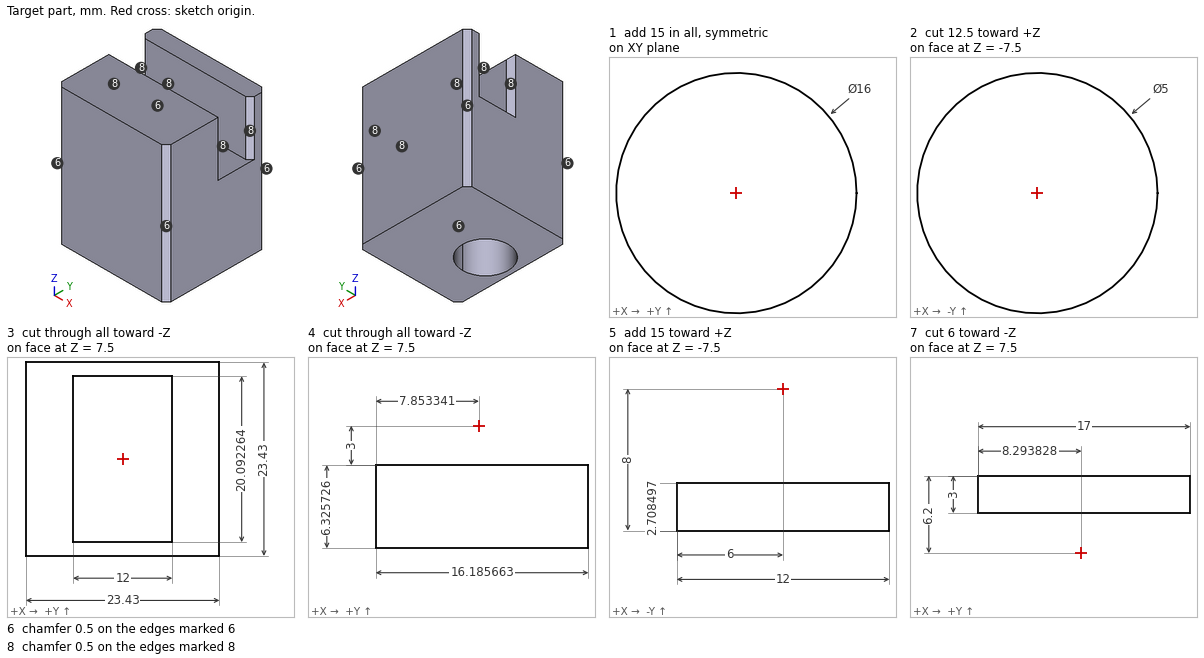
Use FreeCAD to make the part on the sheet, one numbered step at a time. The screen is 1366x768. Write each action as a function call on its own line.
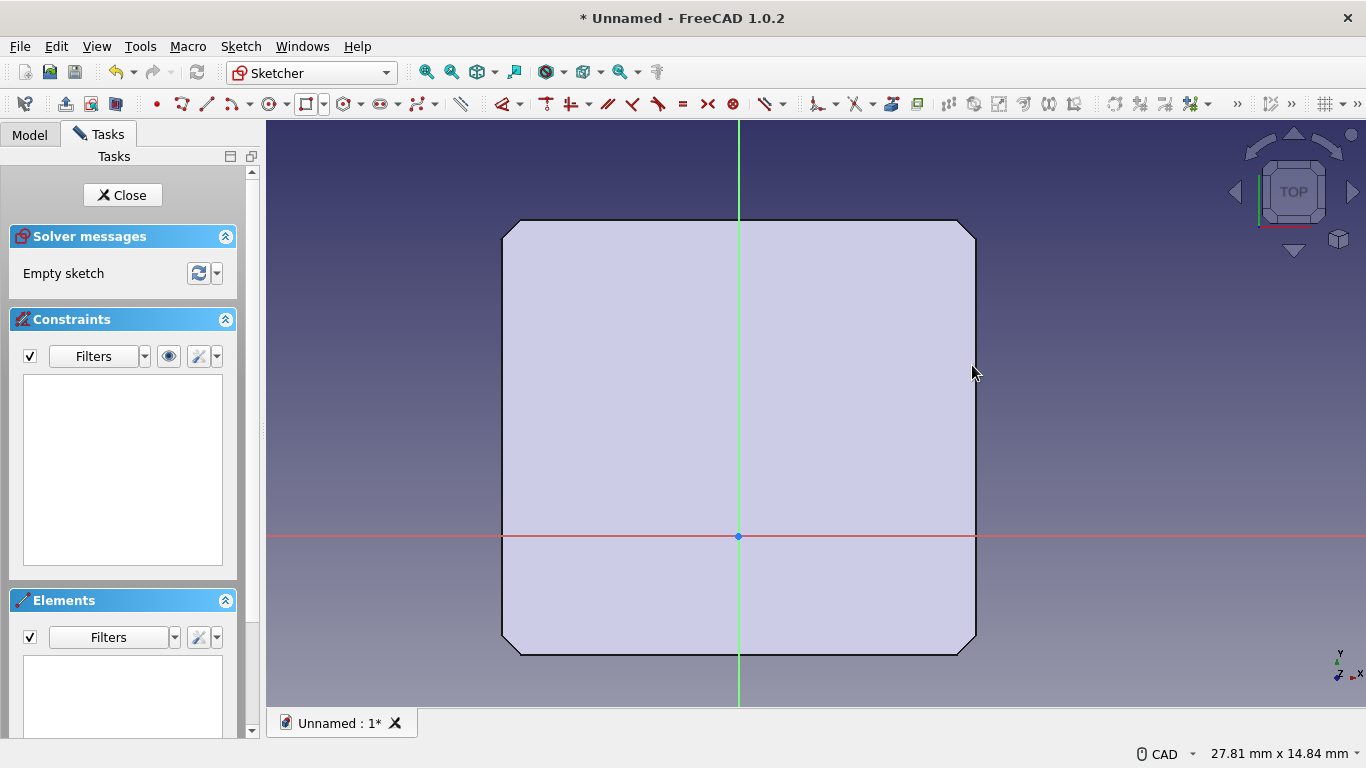
click(306, 104)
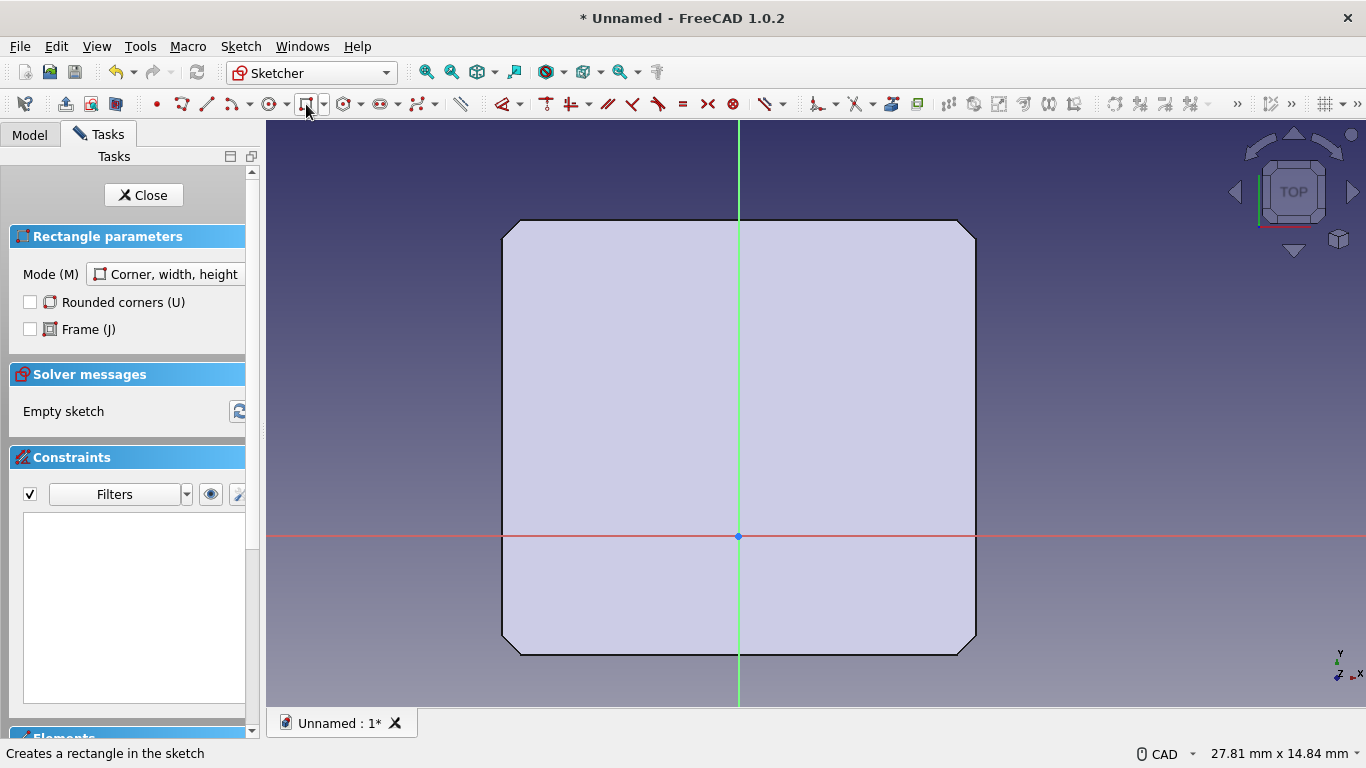
click(411, 291)
click(1083, 409)
key(Escape)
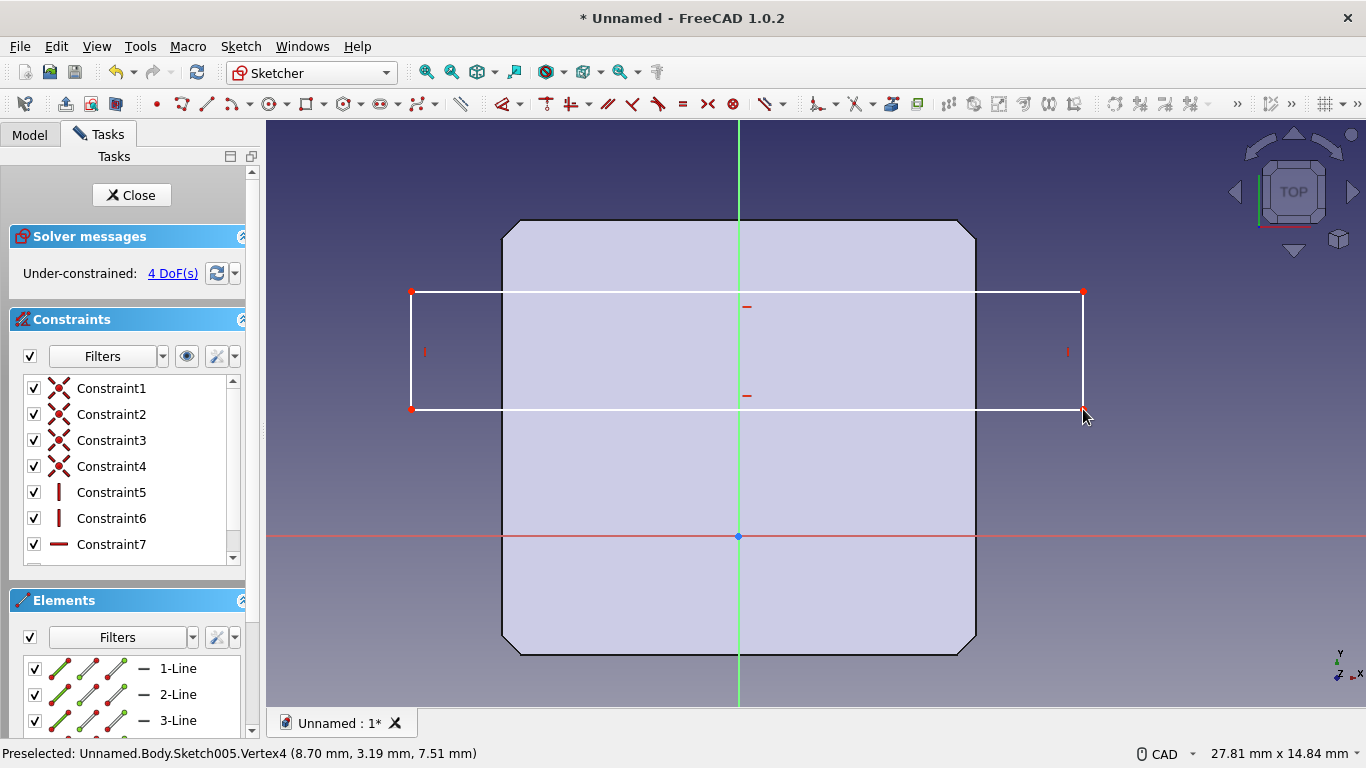
click(502, 104)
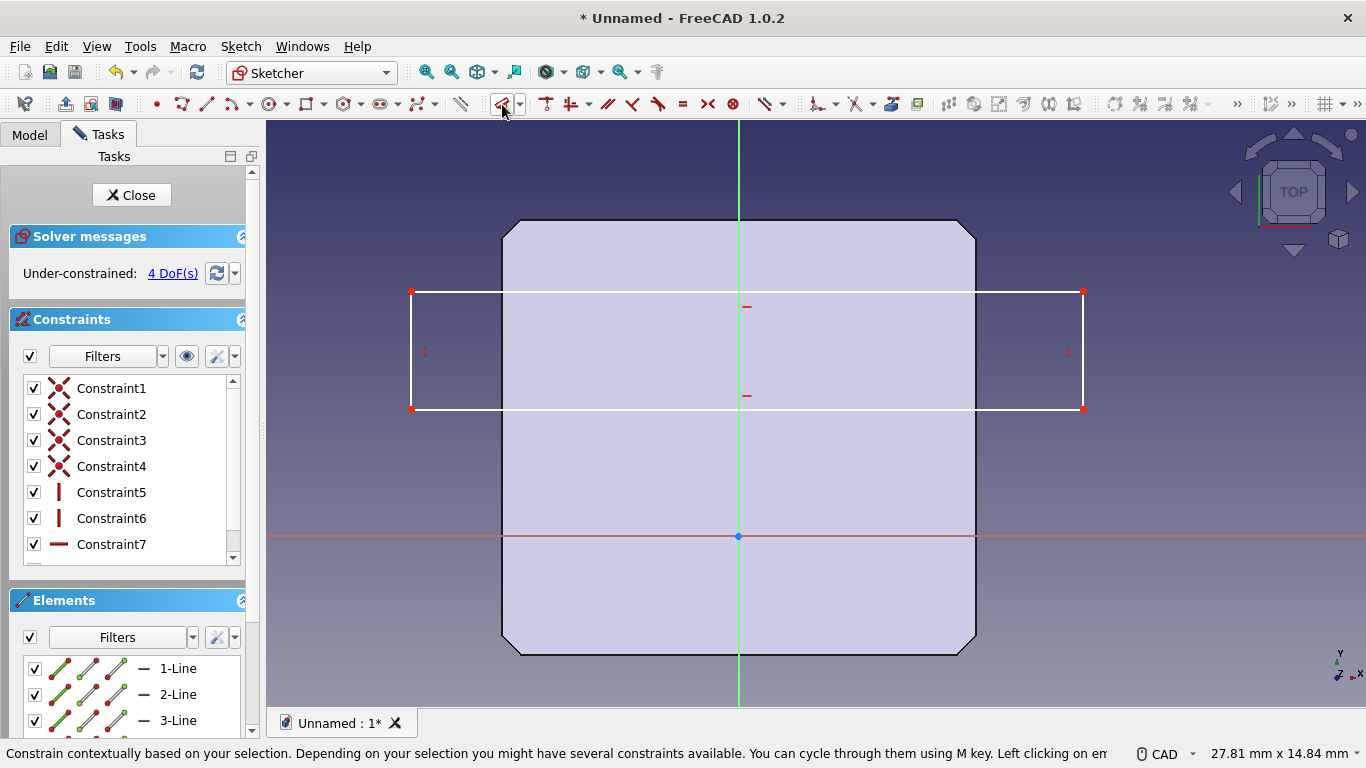
click(411, 327)
click(377, 351)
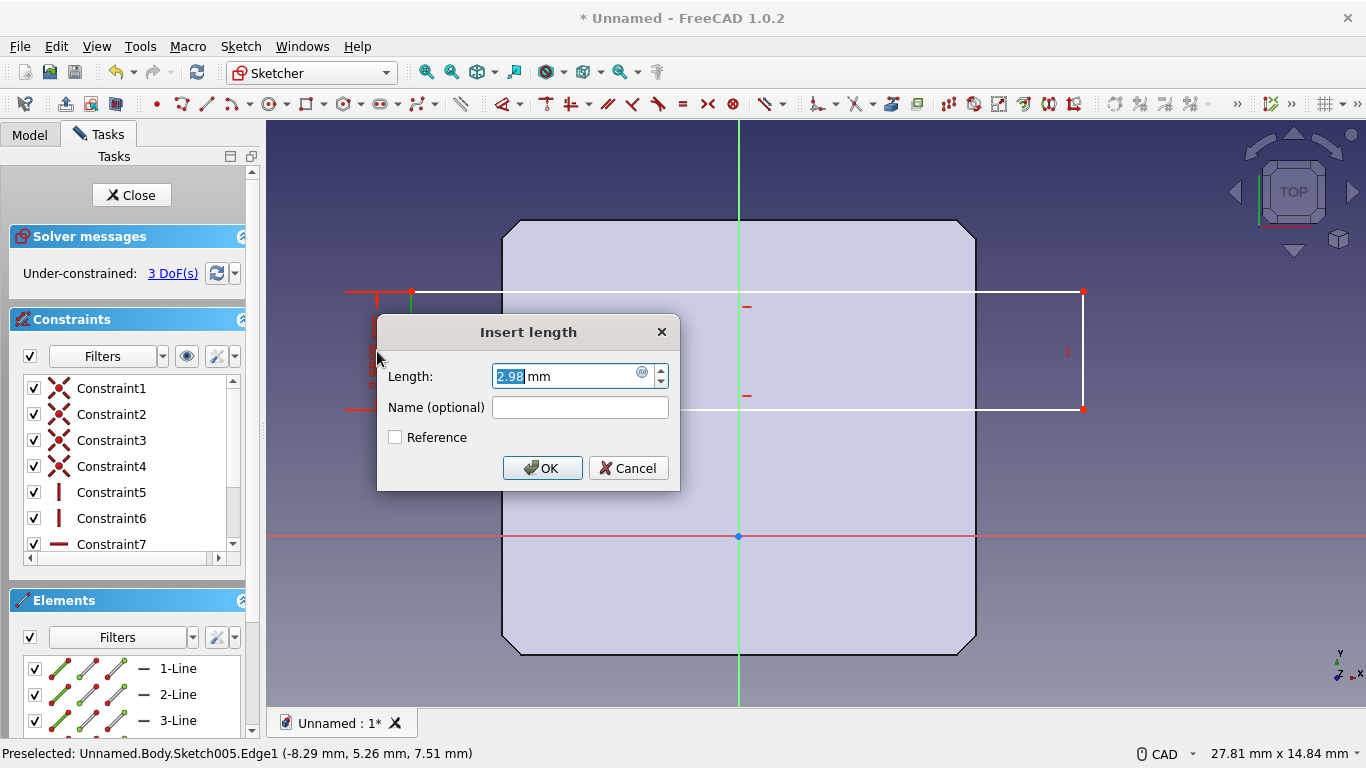
text(3)
key(Return)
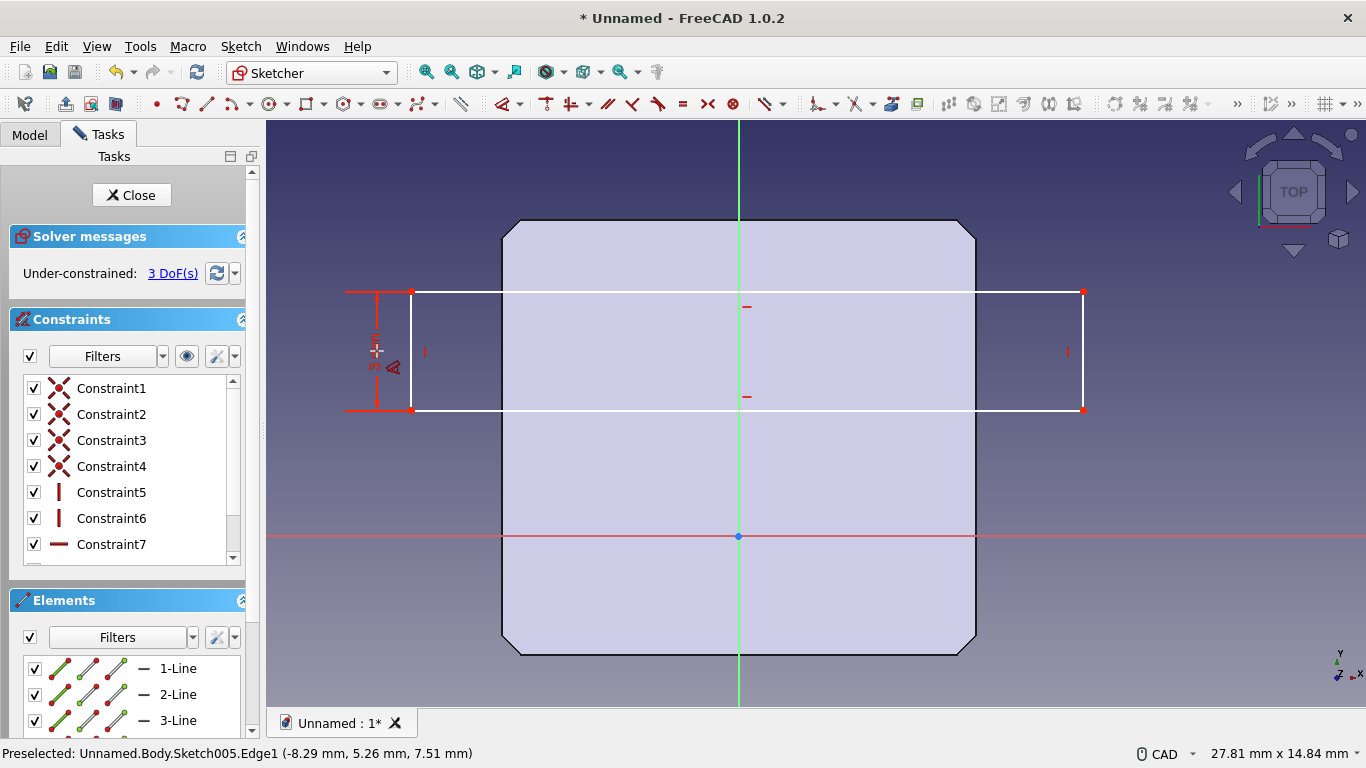
click(613, 411)
click(592, 377)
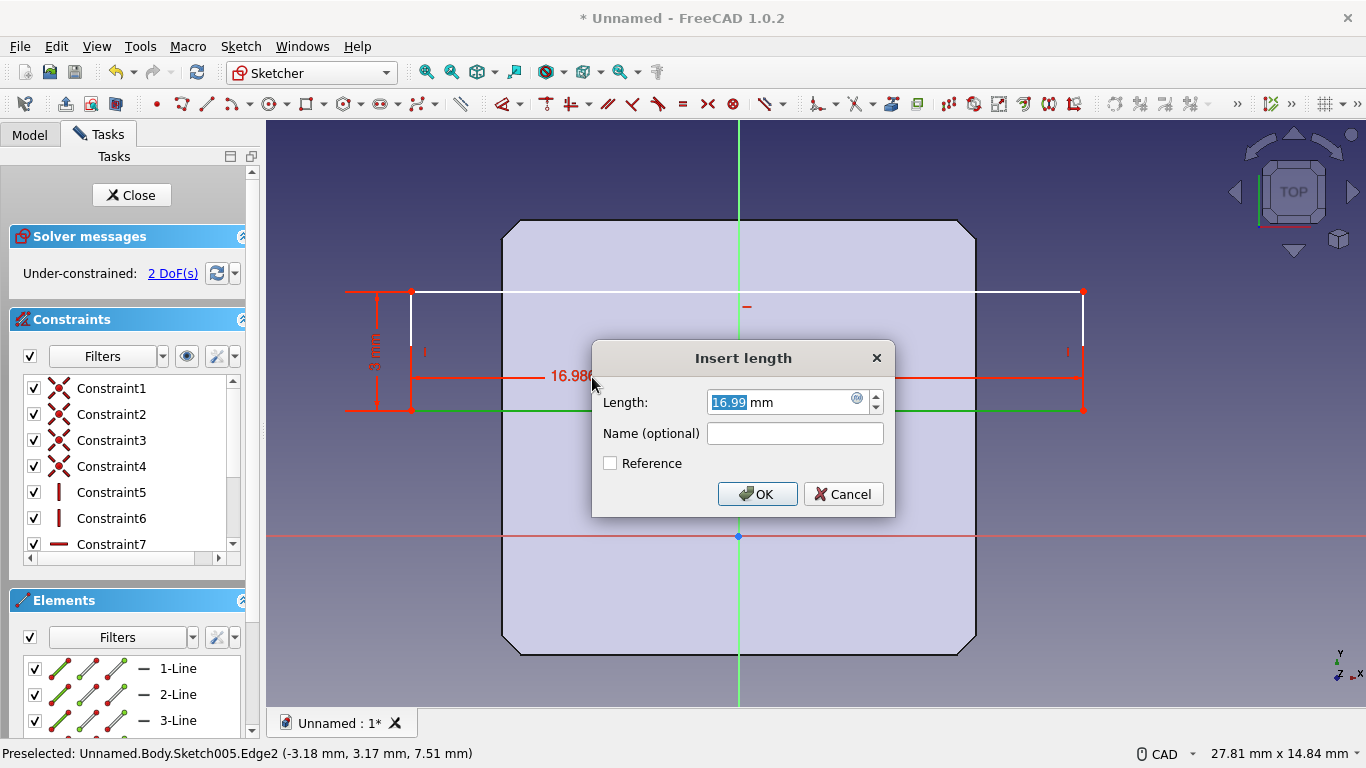
text(17)
key(Return)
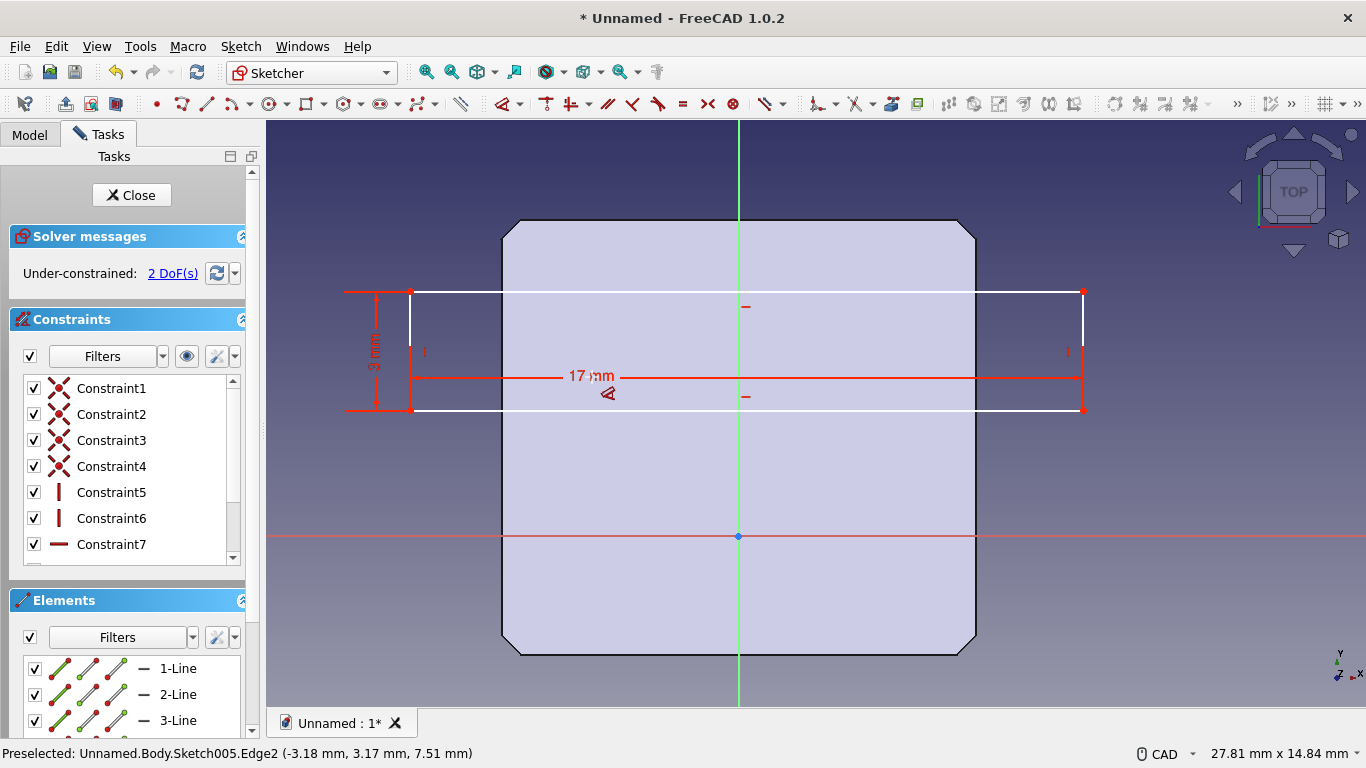
click(410, 292)
click(376, 414)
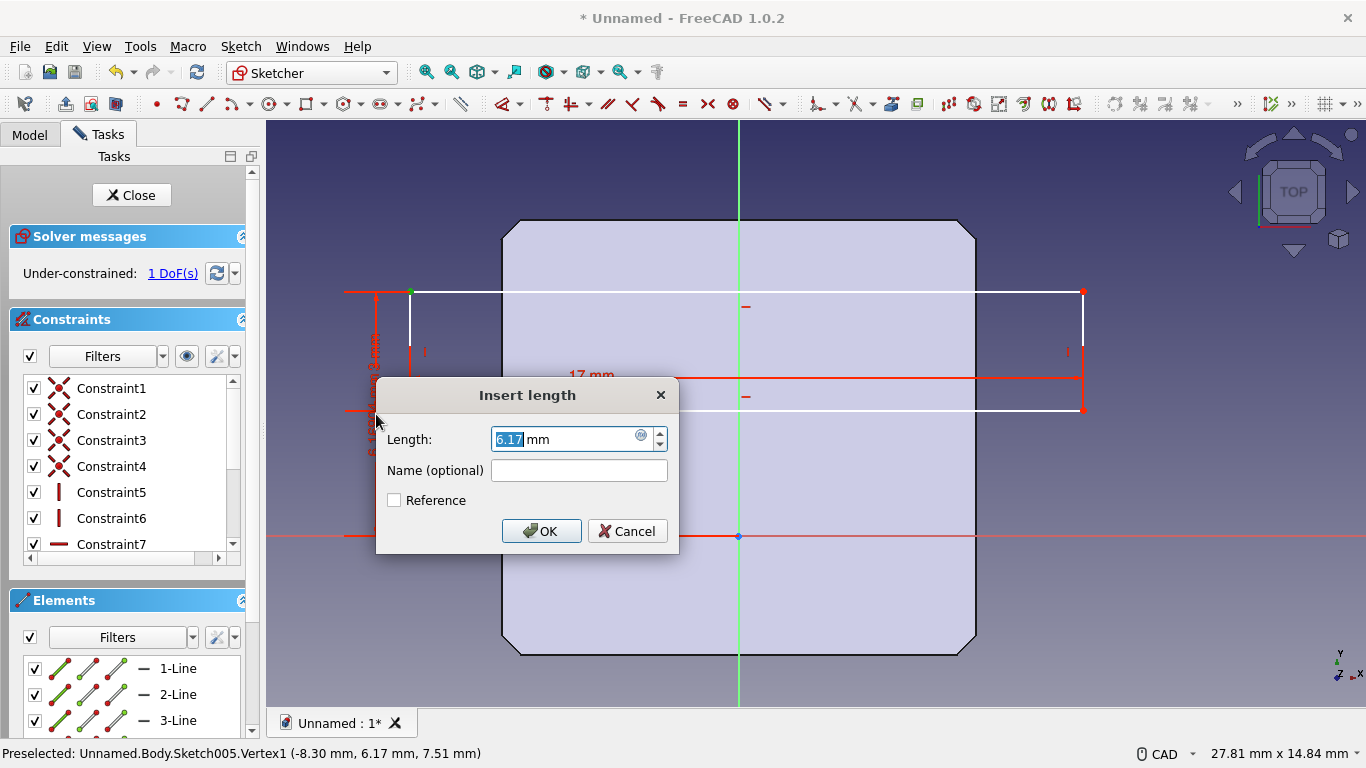
text(6.2)
key(Return)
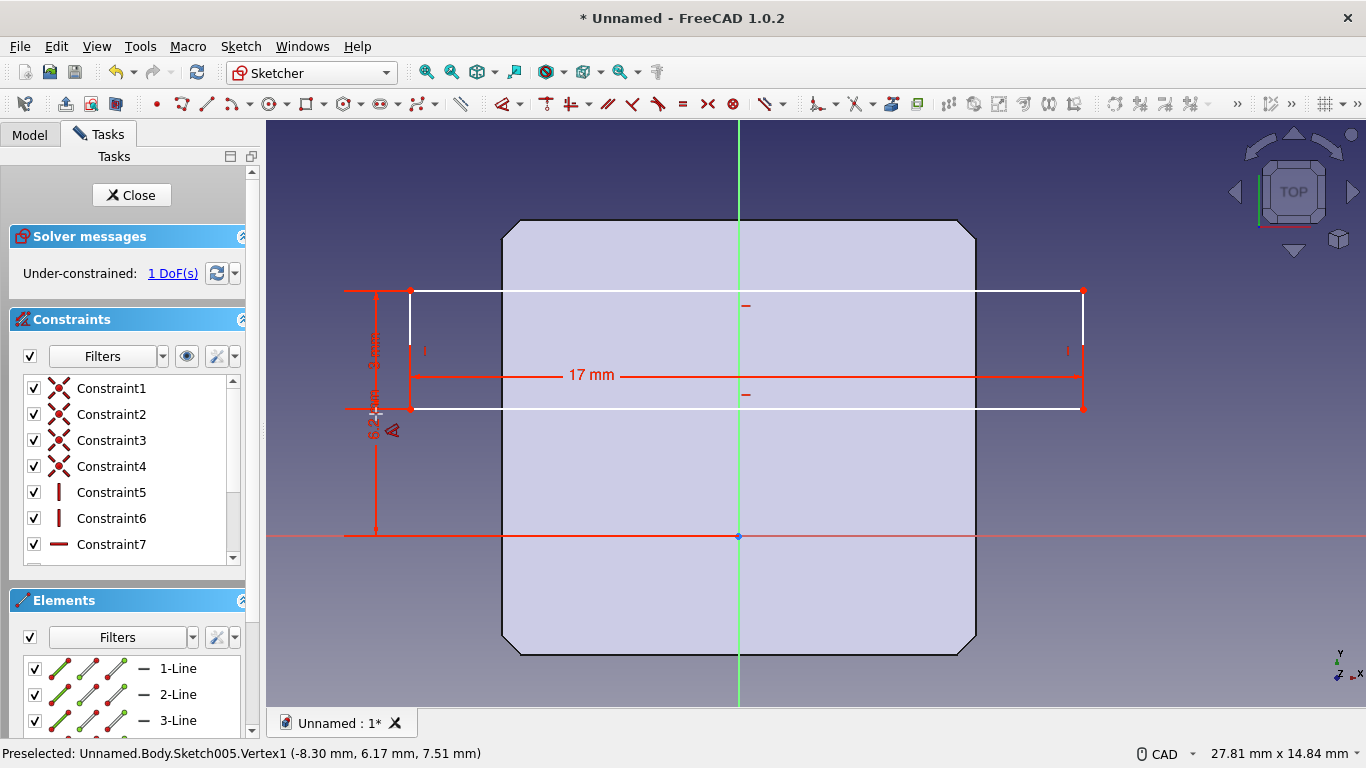
click(410, 291)
click(575, 570)